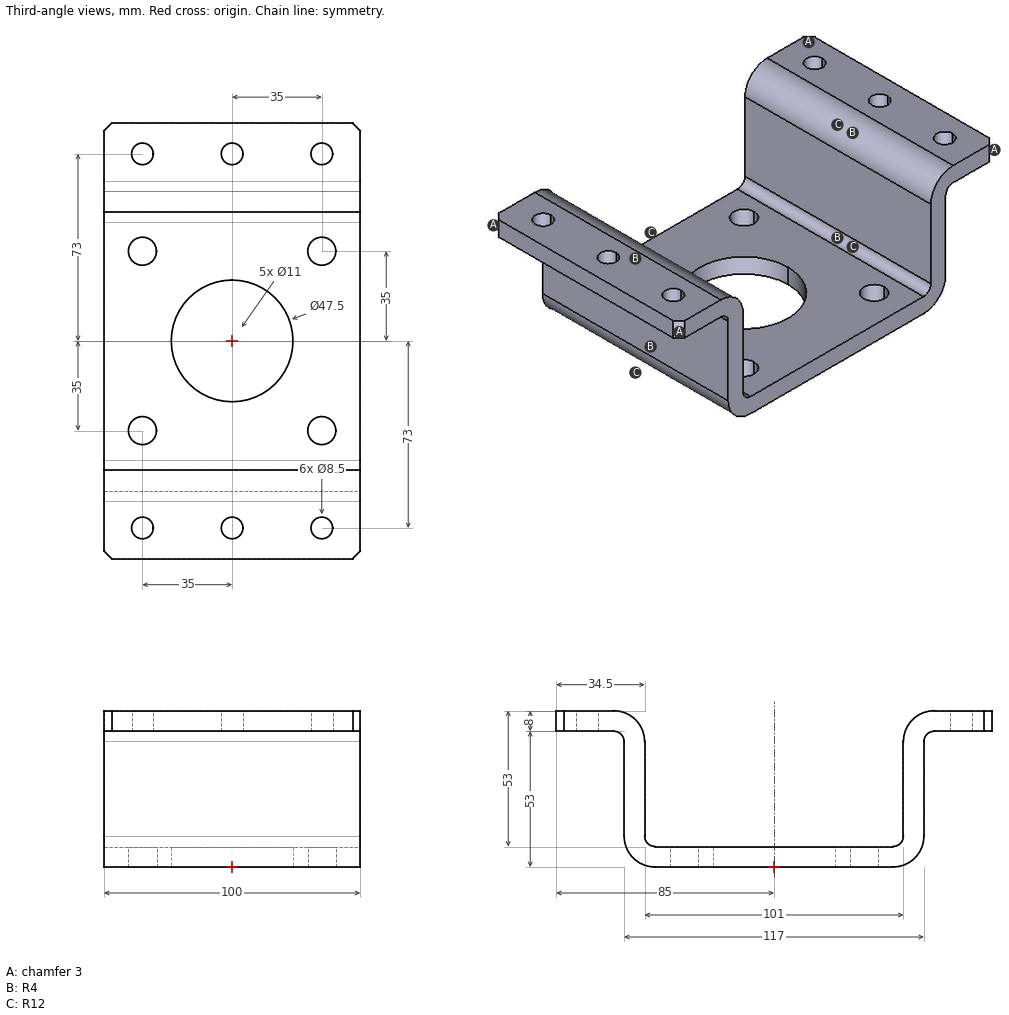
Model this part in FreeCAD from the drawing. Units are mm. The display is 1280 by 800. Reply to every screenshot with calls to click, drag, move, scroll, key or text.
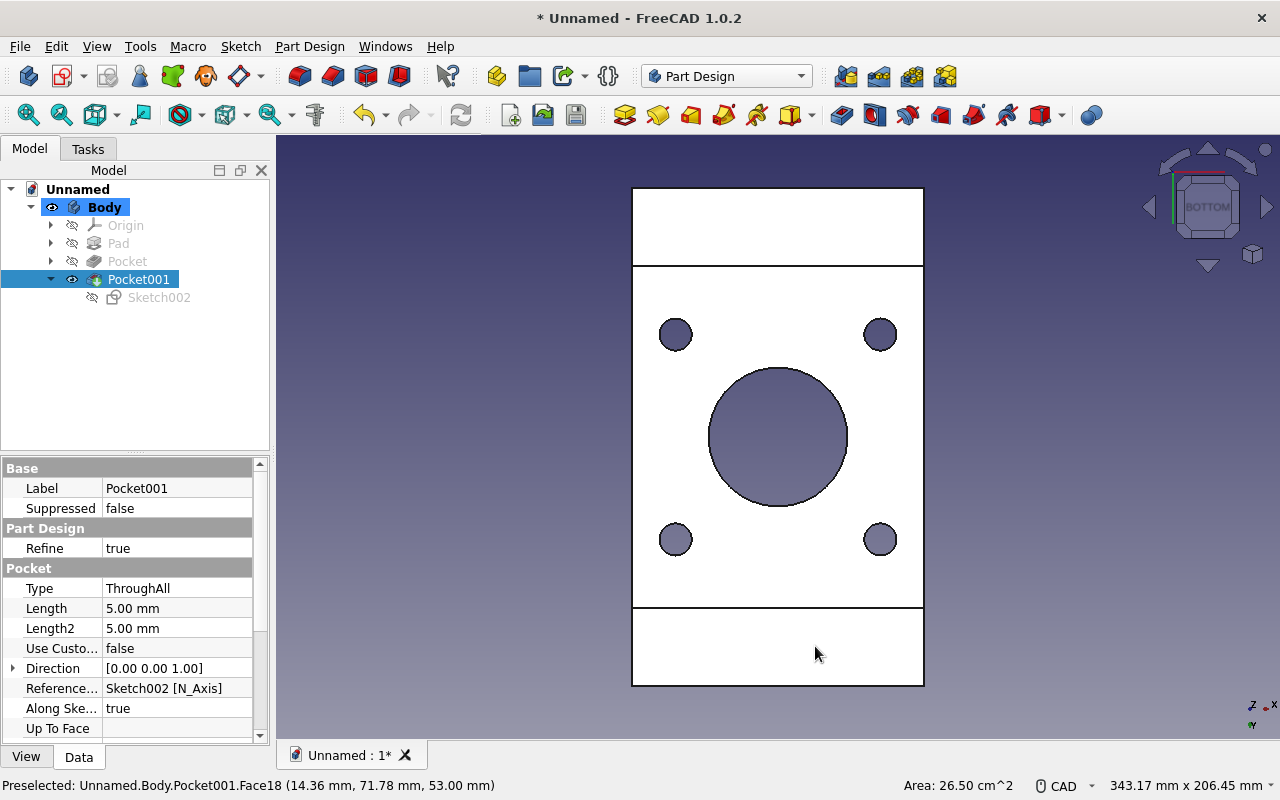
click(62, 76)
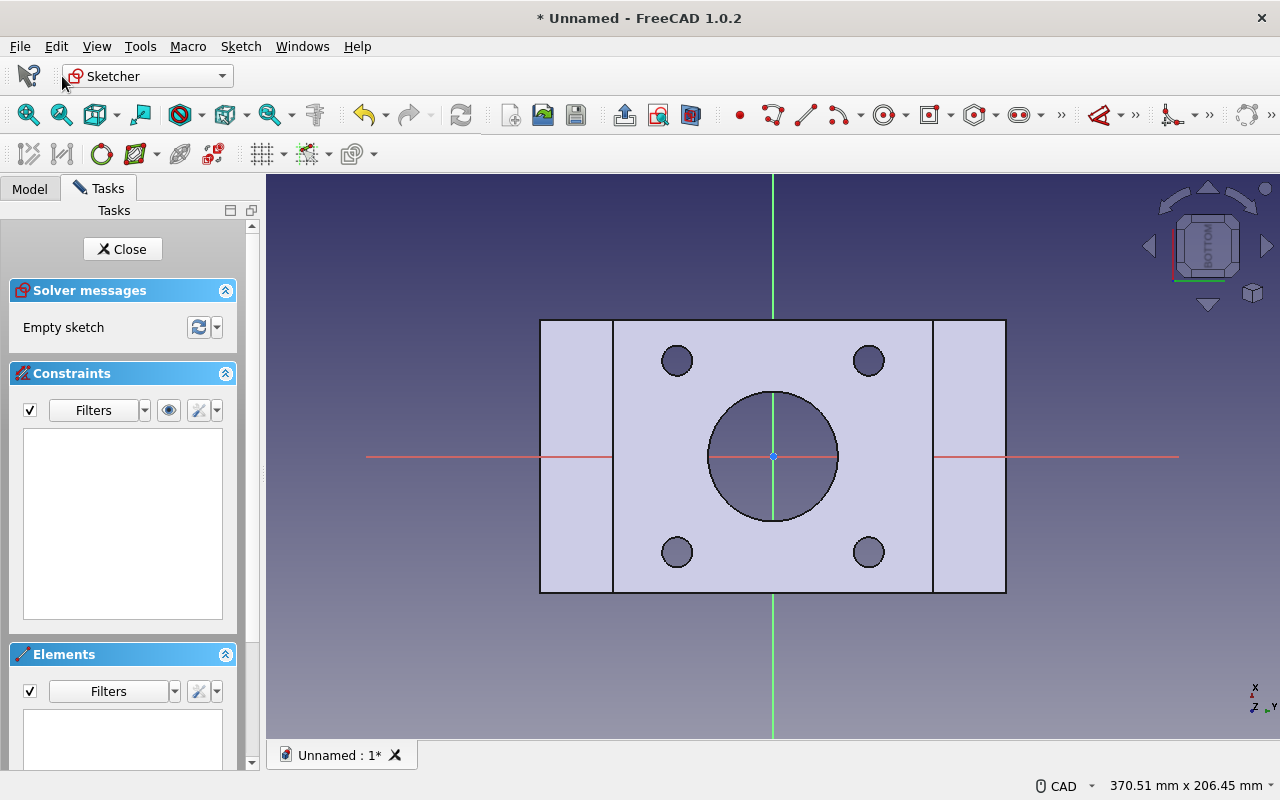
click(691, 116)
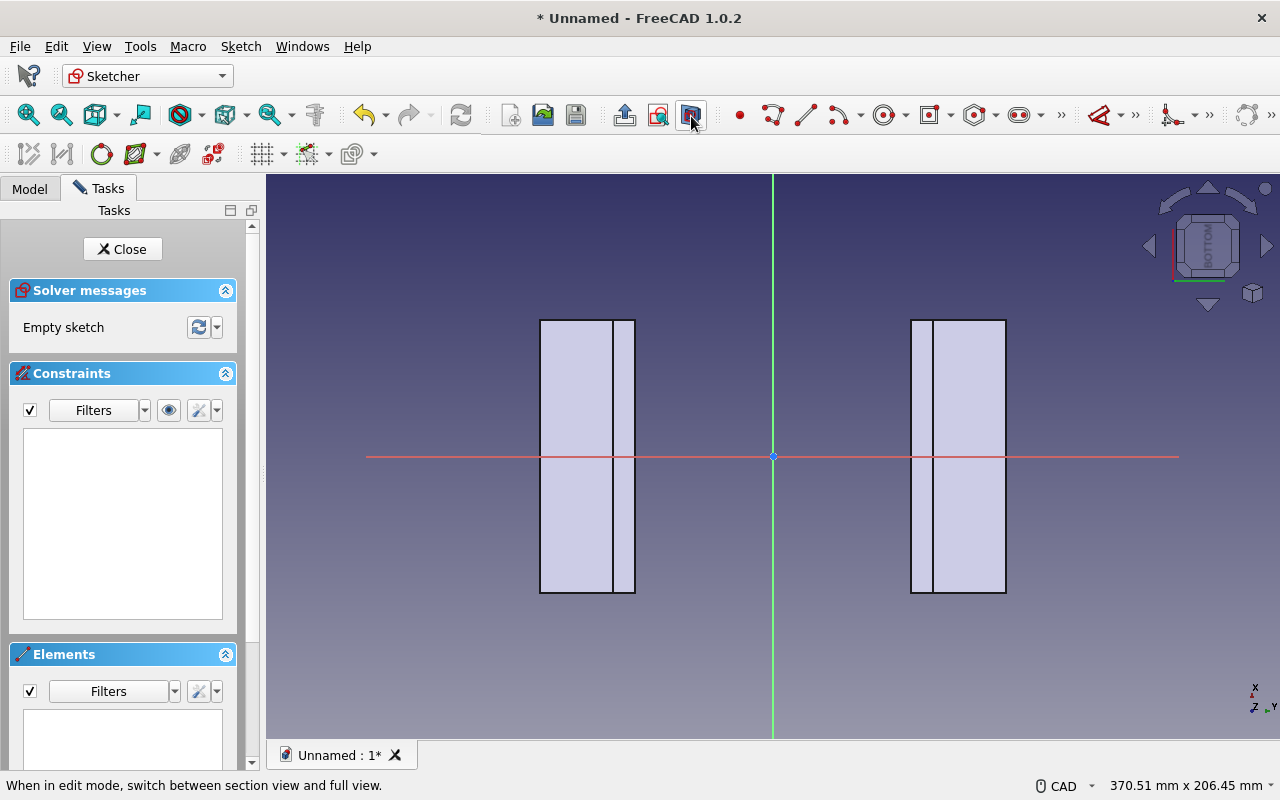
scroll(912, 457, up, 2)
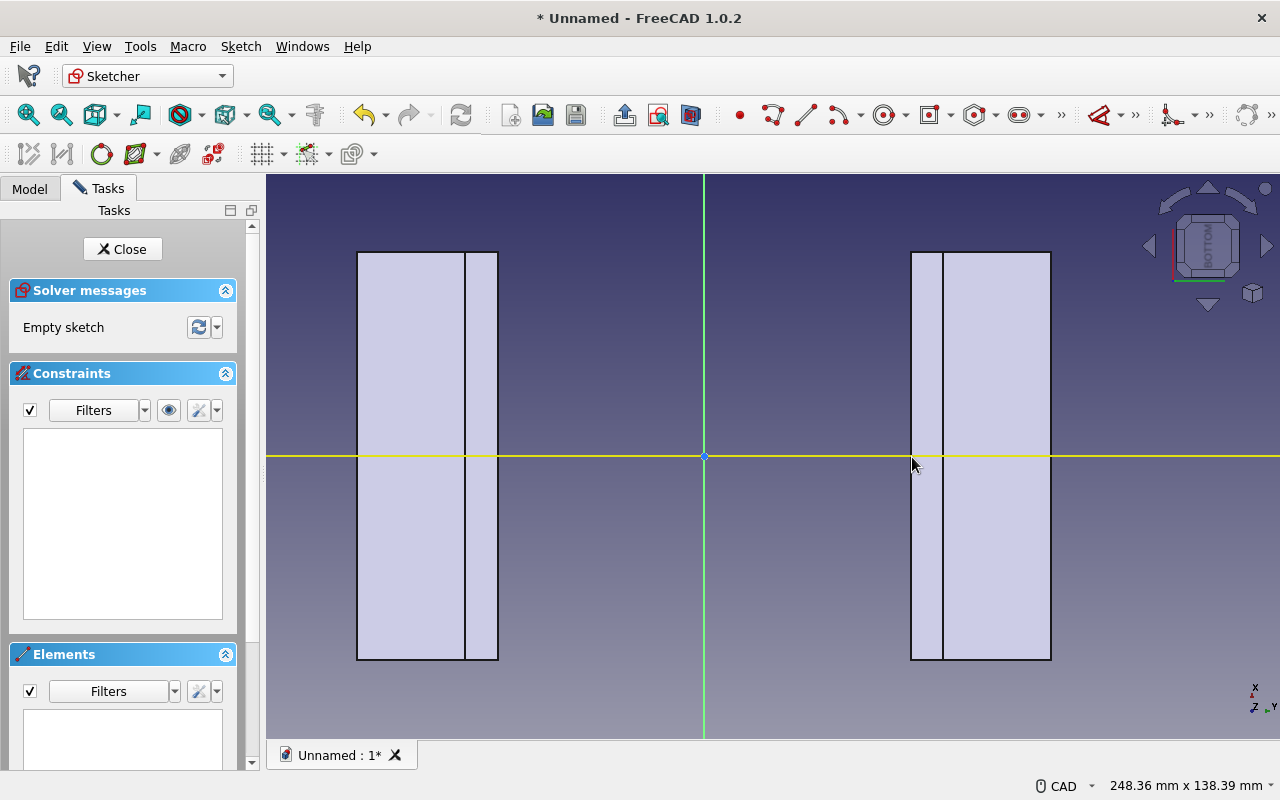
click(884, 116)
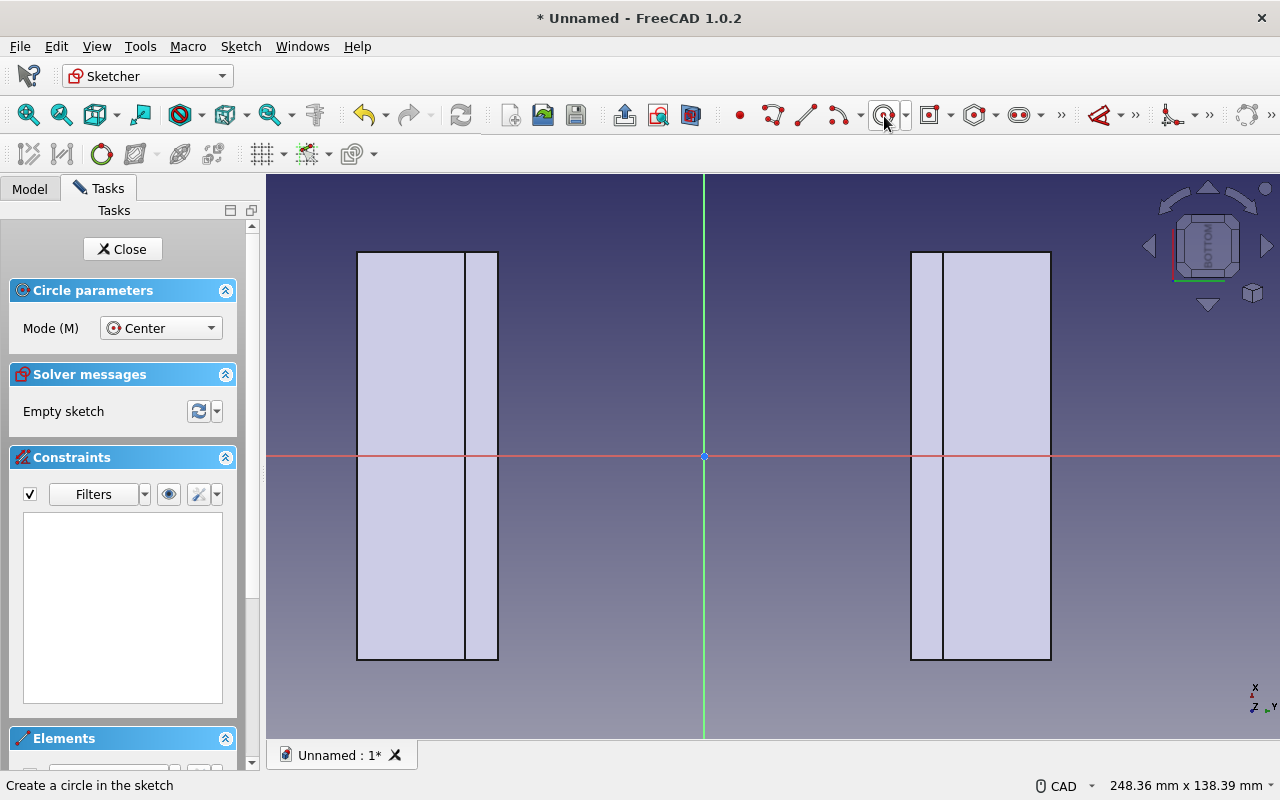
scroll(406, 313, up, 2)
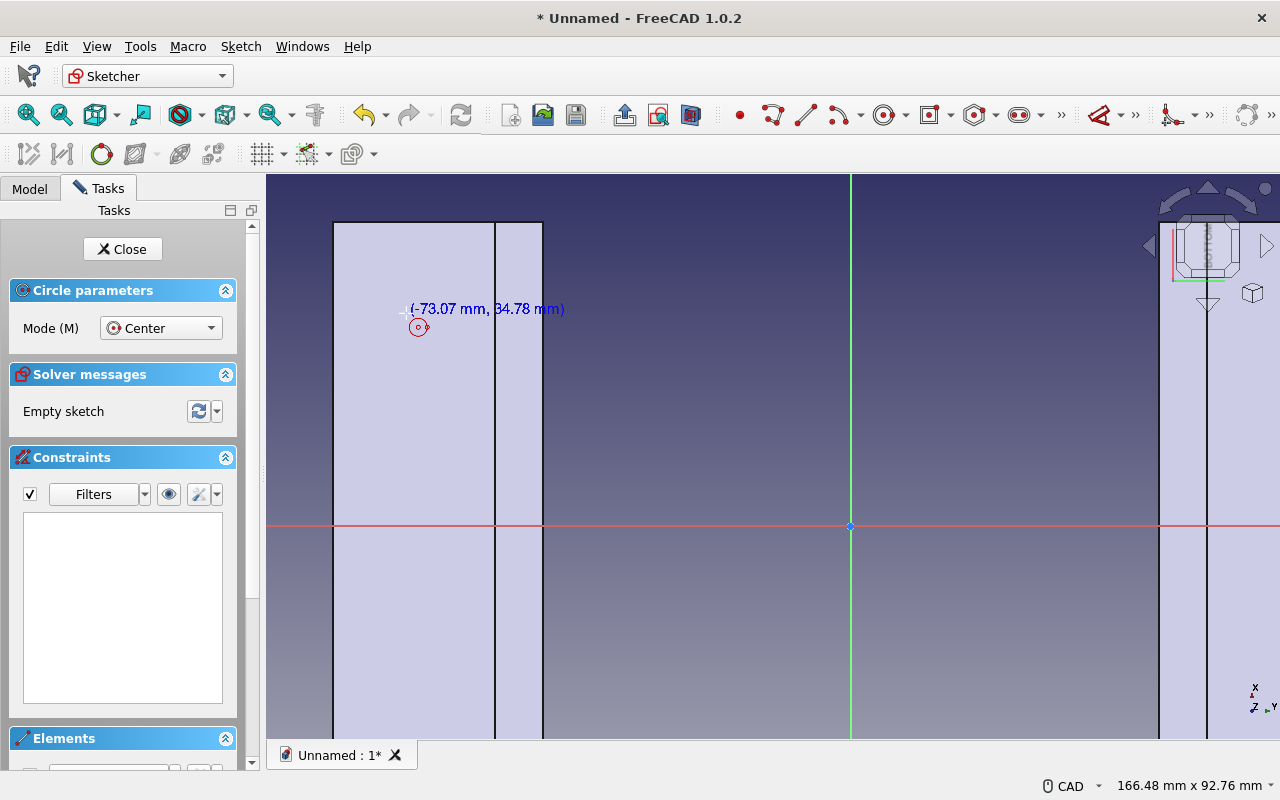
click(406, 313)
move(425, 295)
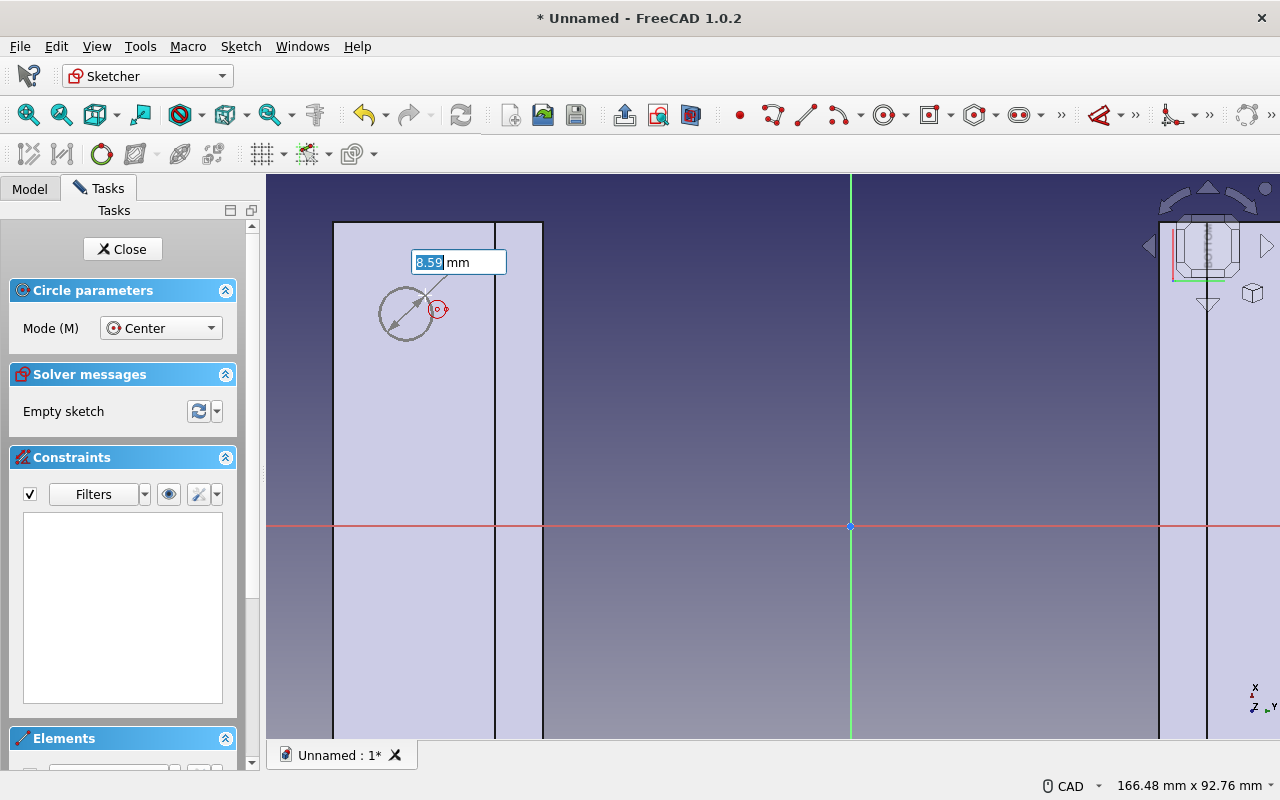
text(8.5)
key(Return)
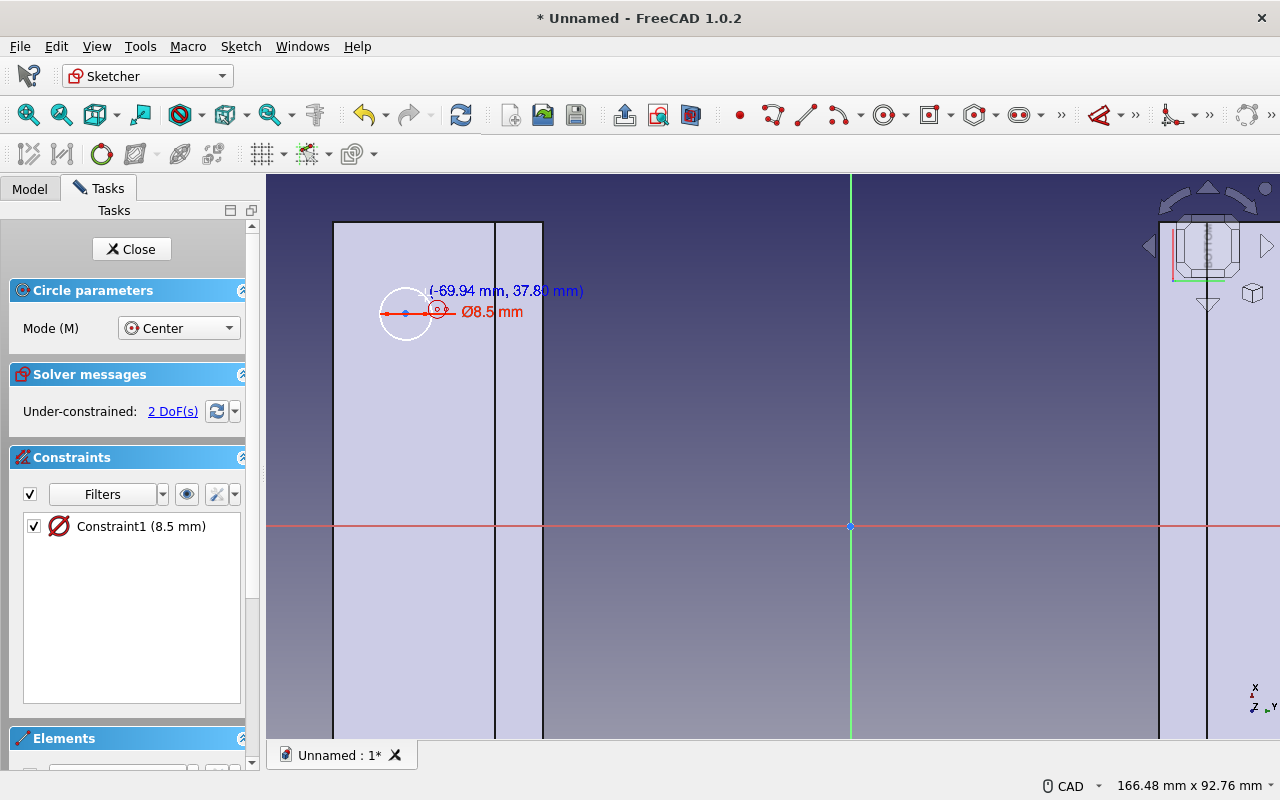
click(406, 526)
move(425, 508)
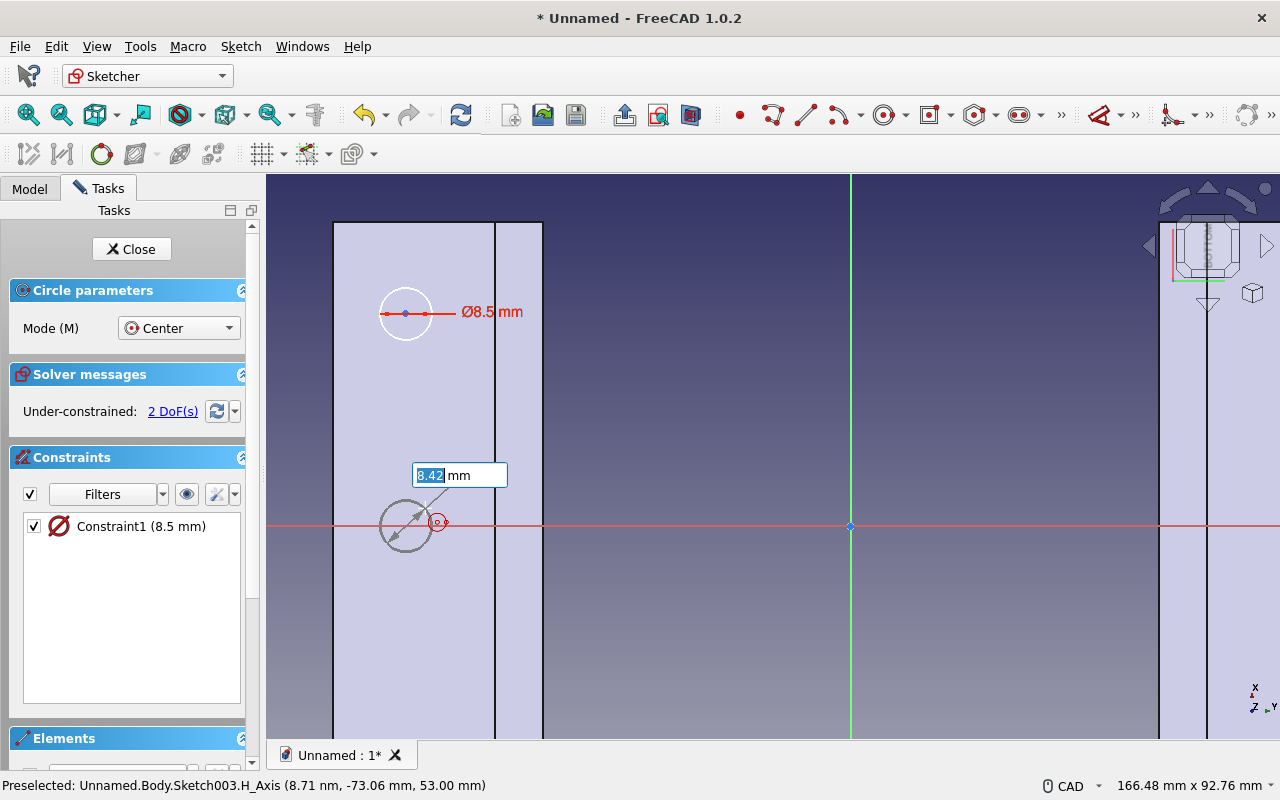
text(8.5)
key(Return)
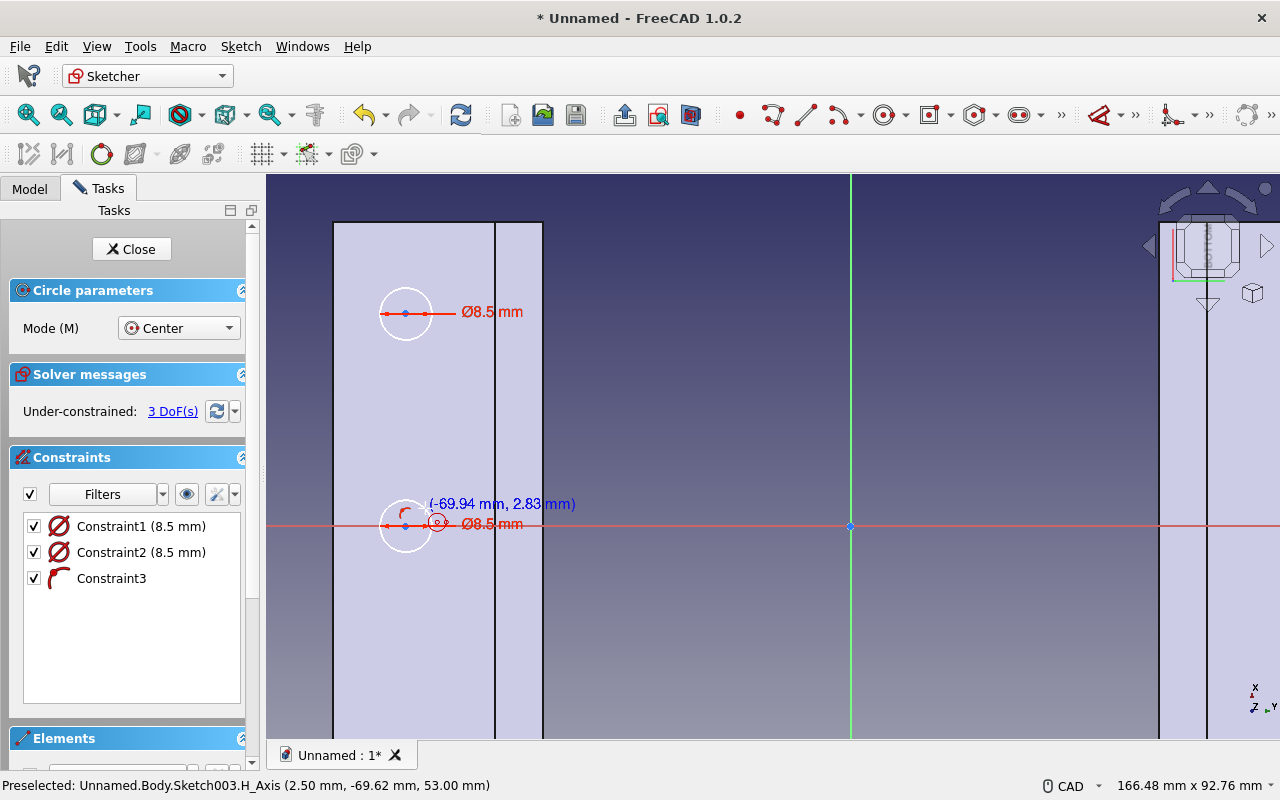
scroll(407, 315, down, 2)